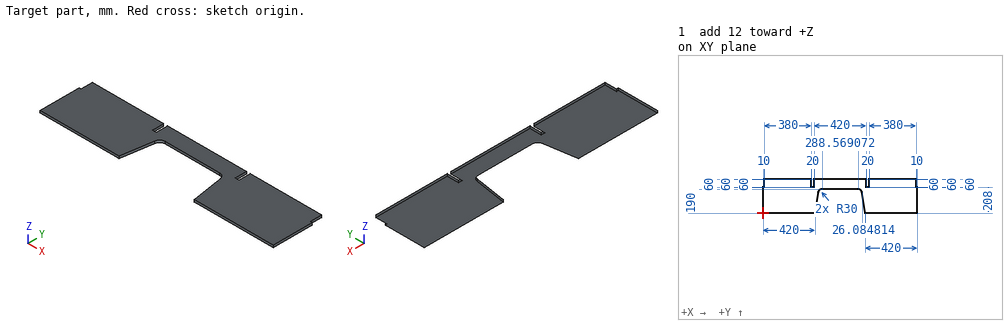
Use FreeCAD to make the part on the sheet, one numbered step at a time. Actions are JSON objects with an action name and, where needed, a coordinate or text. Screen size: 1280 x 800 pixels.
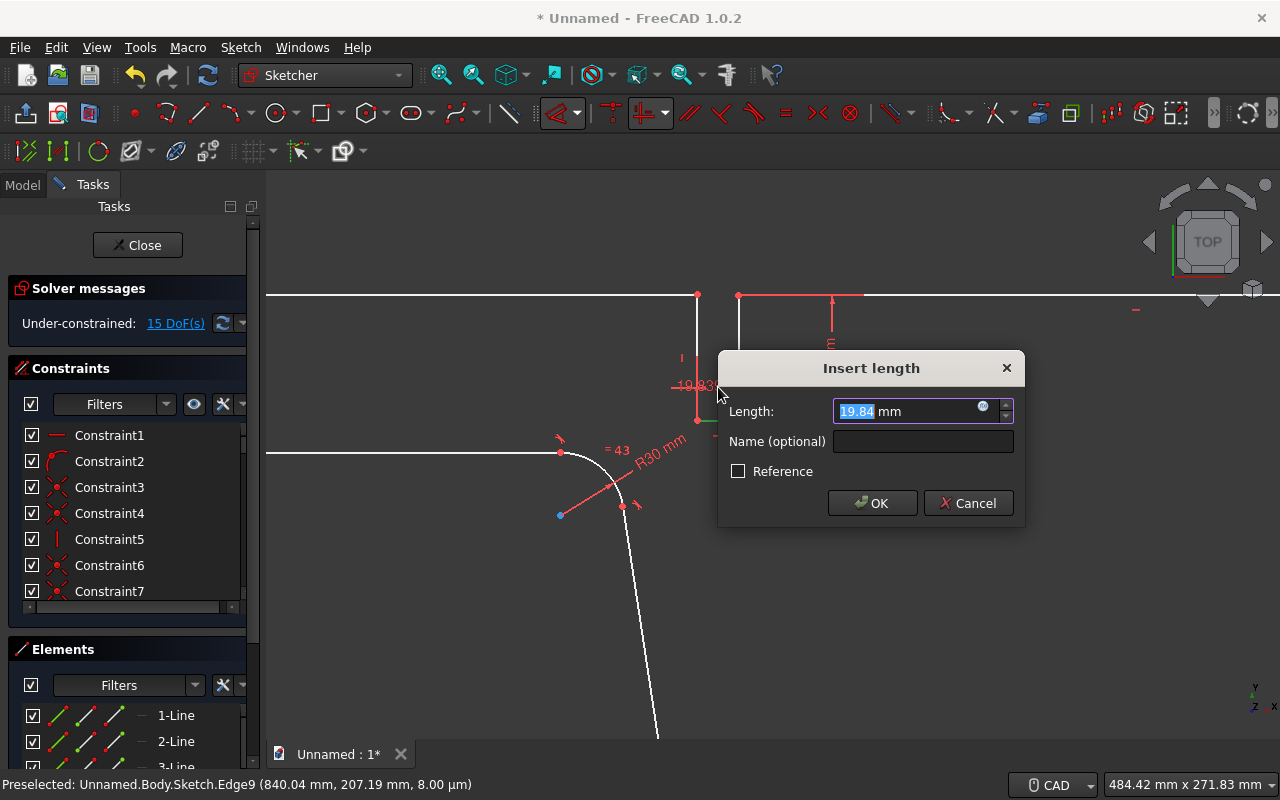
{"action": "type", "text": "20"}
{"action": "key", "text": "Return"}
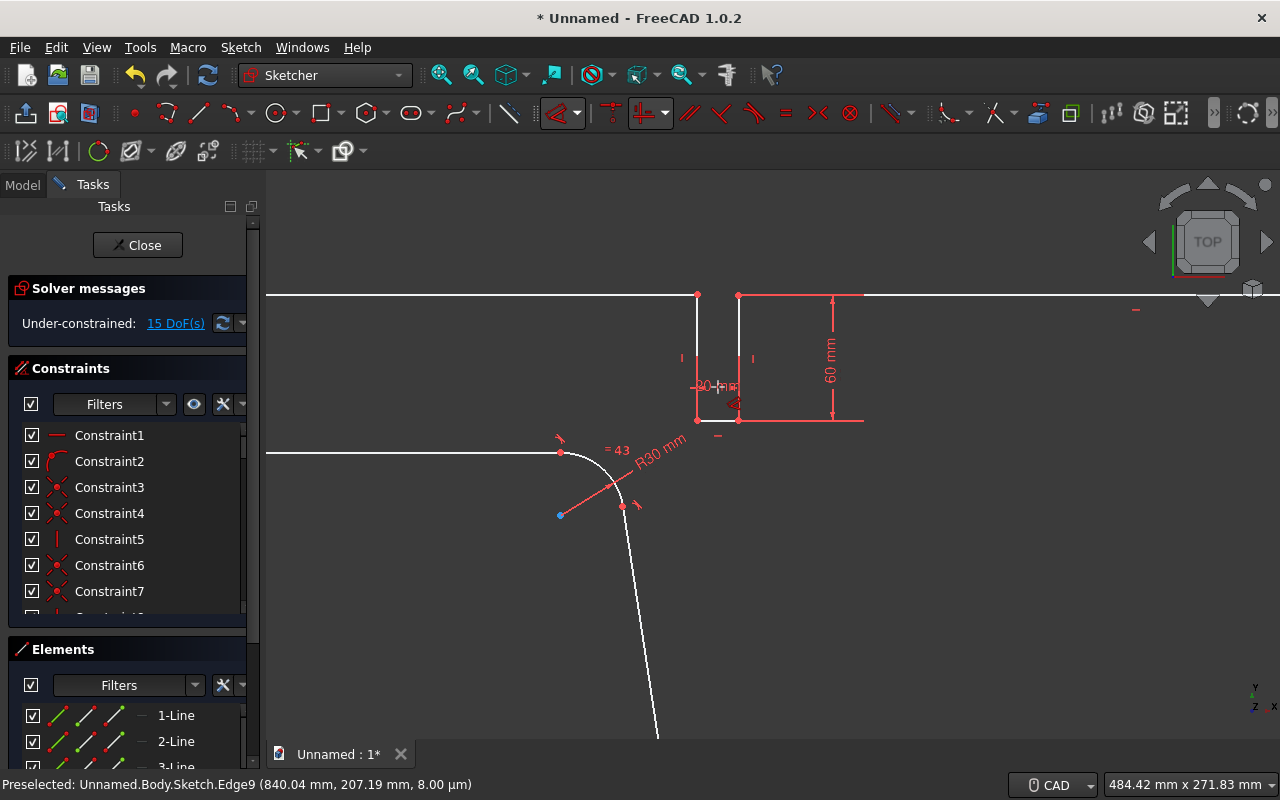
{"action": "left_click", "coordinate": [697, 383]}
{"action": "left_click", "coordinate": [663, 358]}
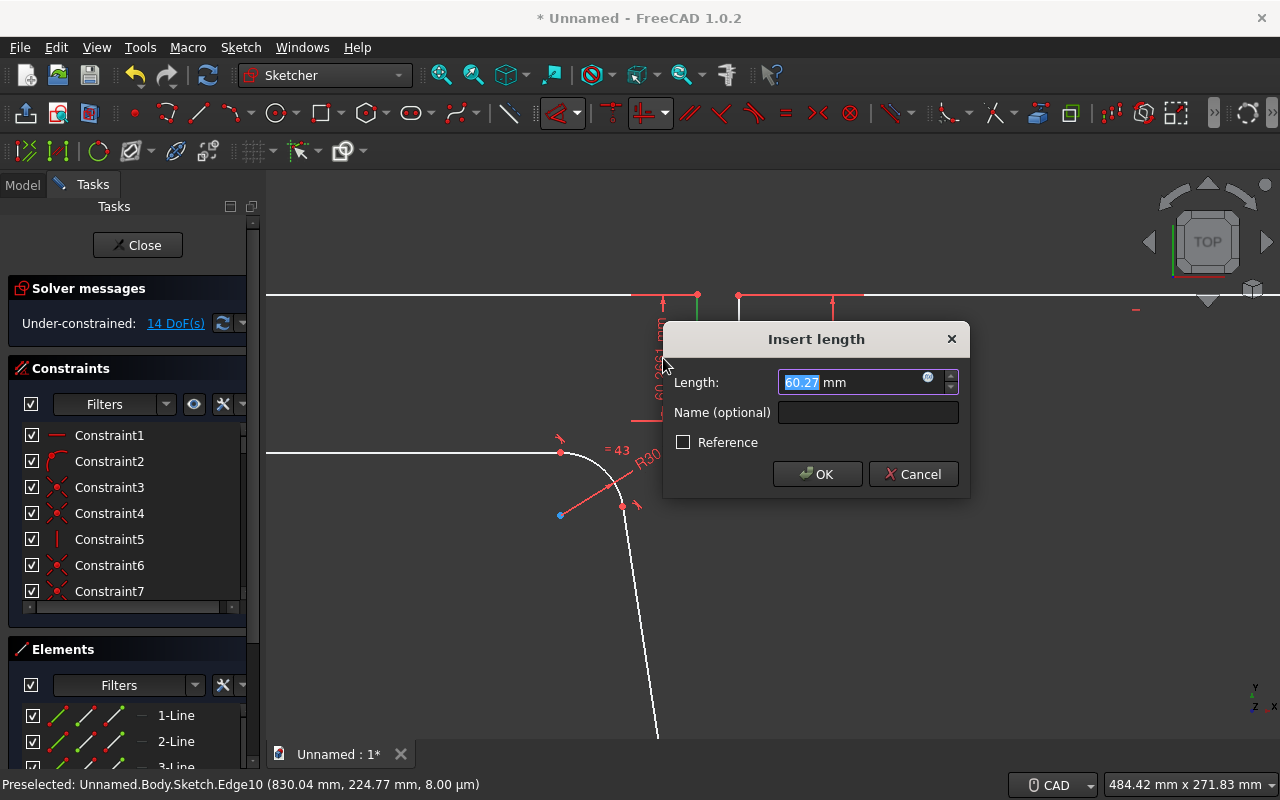
{"action": "type", "text": "60"}
{"action": "key", "text": "Return"}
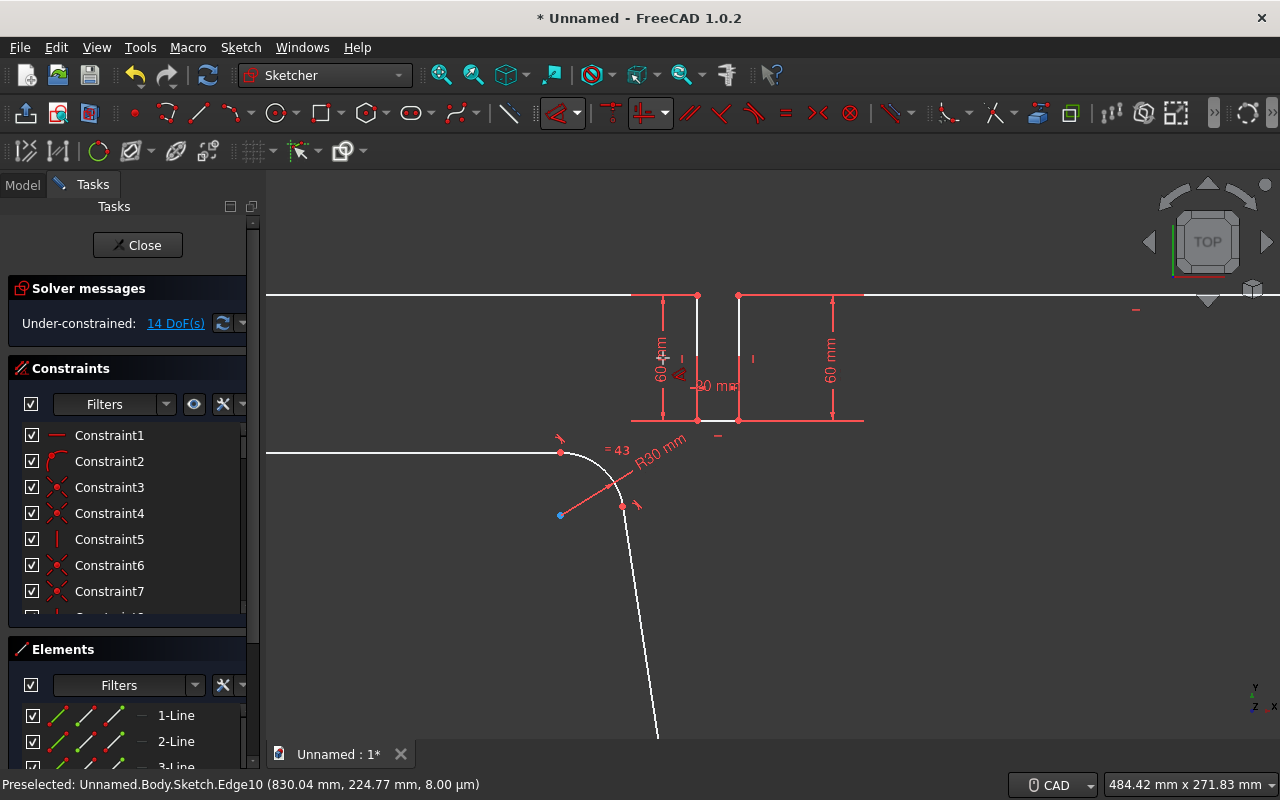
{"action": "scroll", "coordinate": [851, 415], "scroll_direction": "down", "scroll_amount": 7}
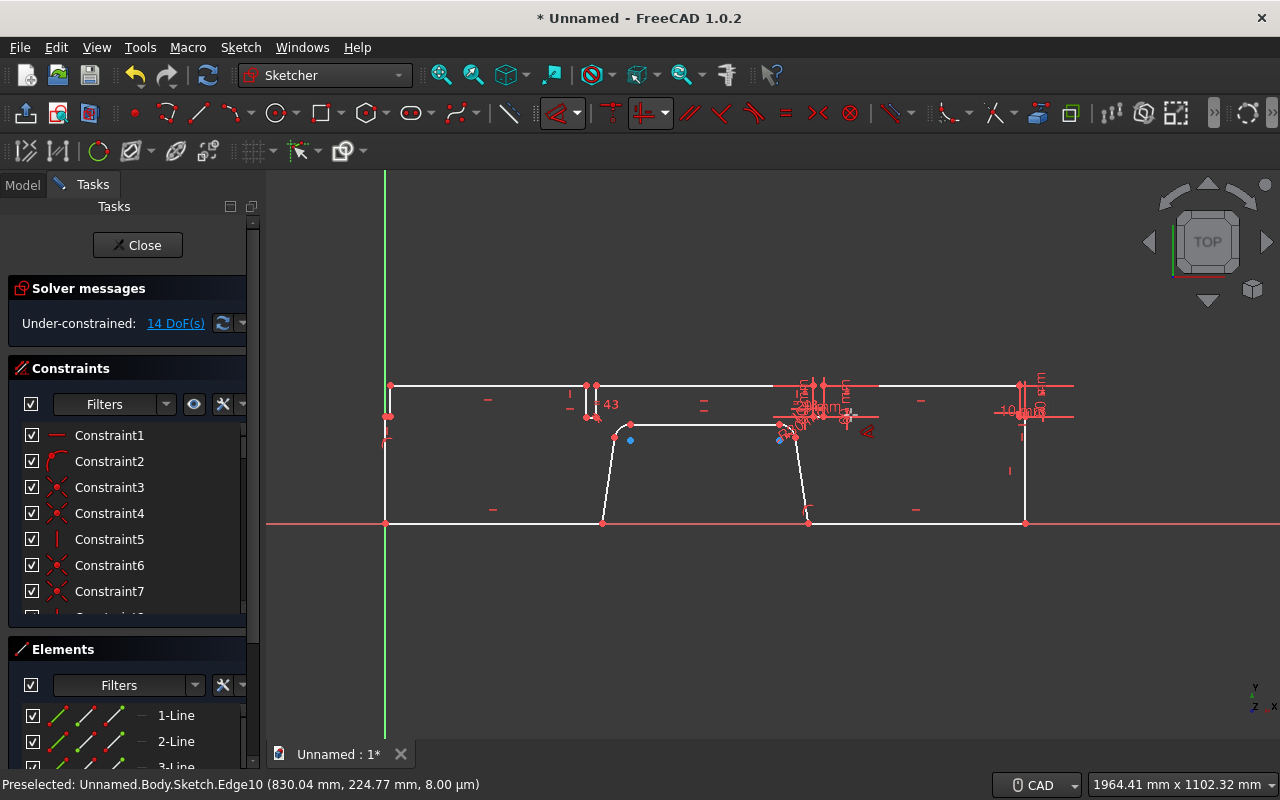
{"action": "scroll", "coordinate": [596, 395], "scroll_direction": "up", "scroll_amount": 2}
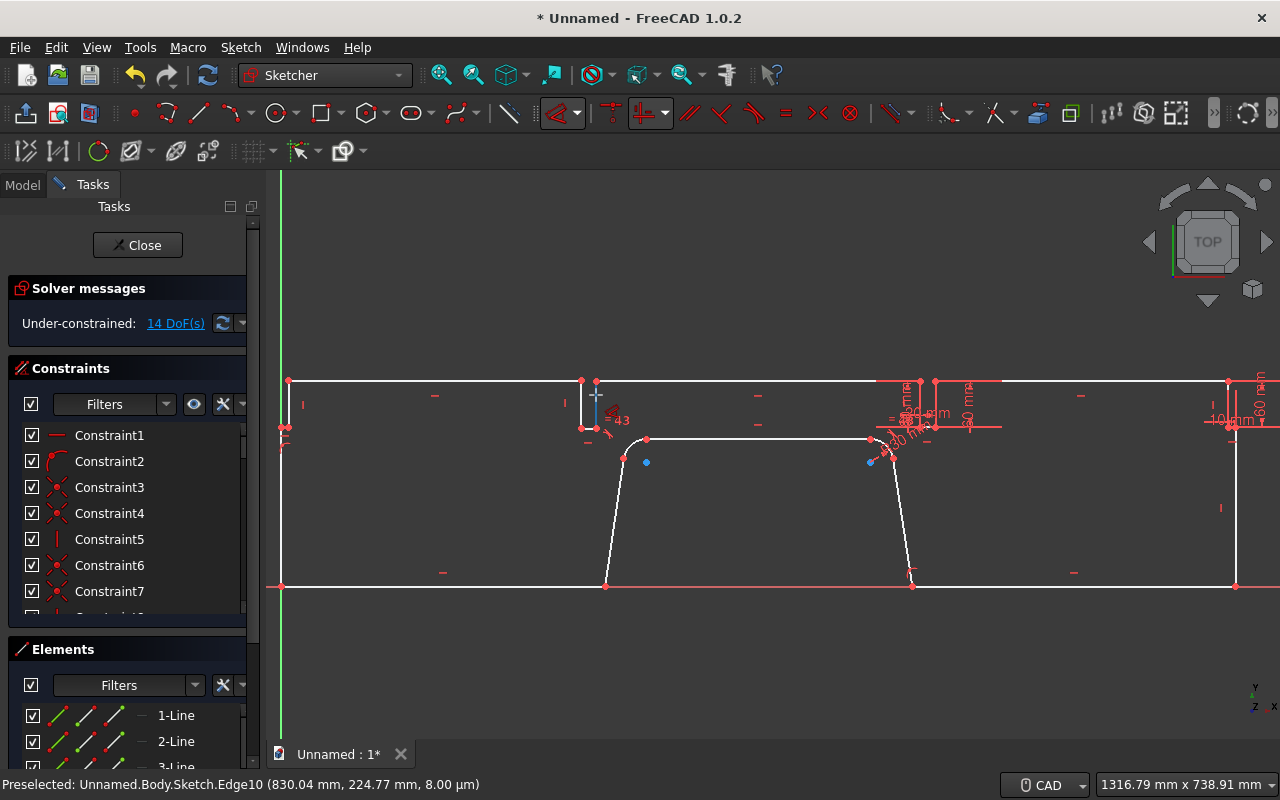
{"action": "left_click", "coordinate": [596, 395]}
{"action": "left_click", "coordinate": [562, 405]}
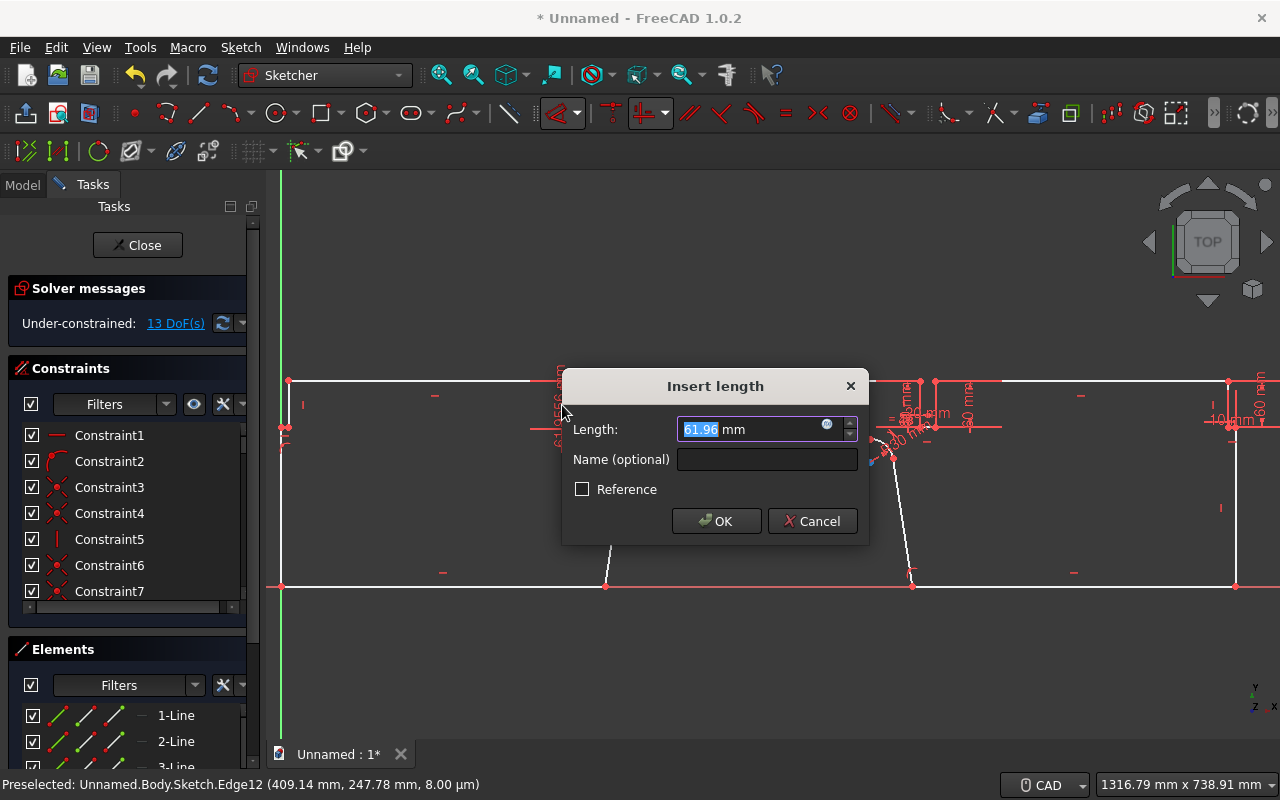
{"action": "type", "text": "60"}
{"action": "key", "text": "Return"}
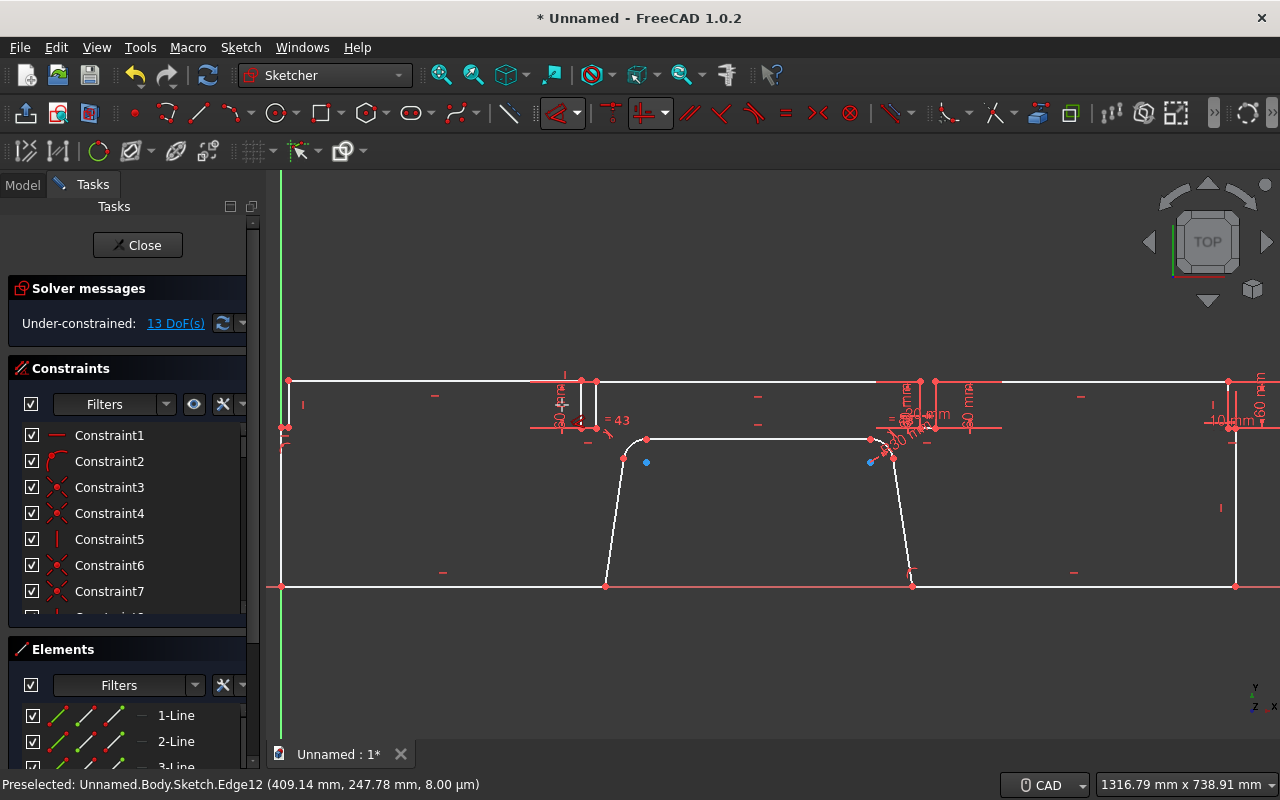
{"action": "scroll", "coordinate": [589, 428], "scroll_direction": "up", "scroll_amount": 5}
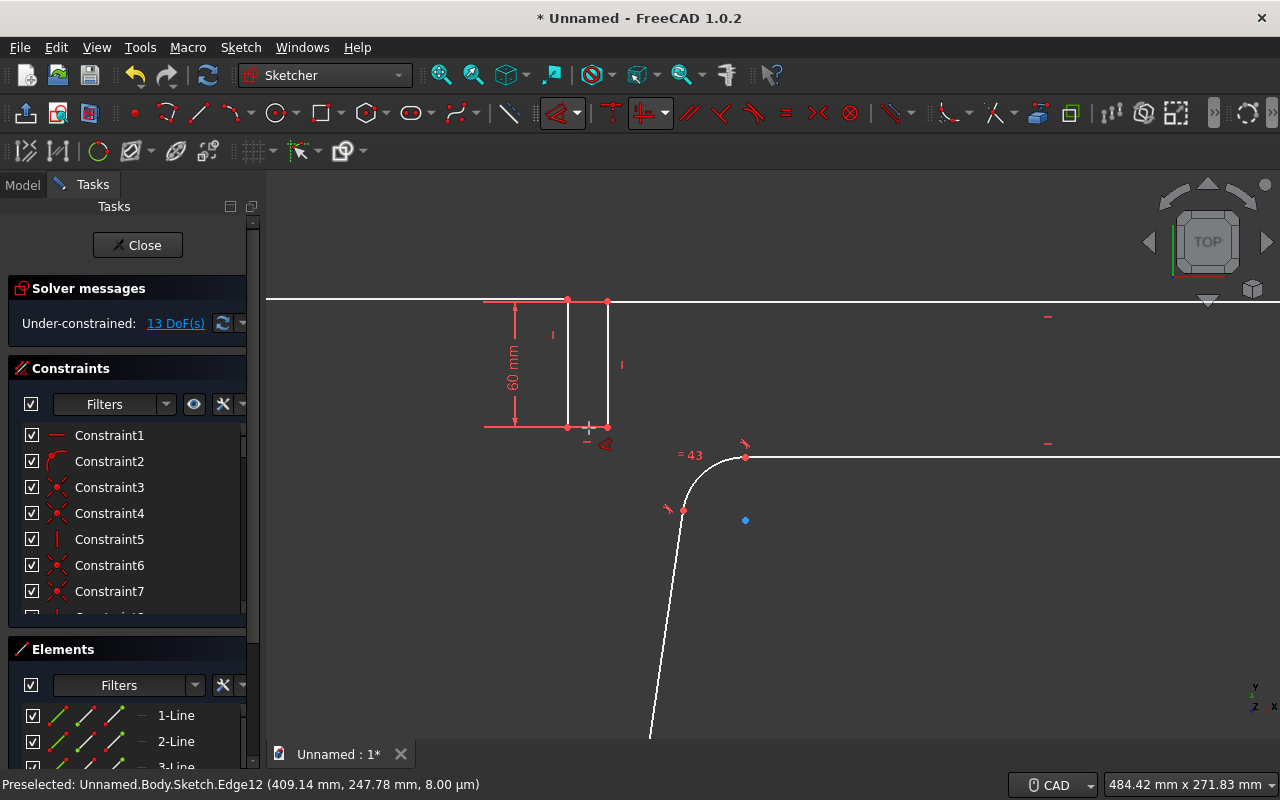
{"action": "left_click", "coordinate": [588, 427]}
{"action": "left_click", "coordinate": [588, 393]}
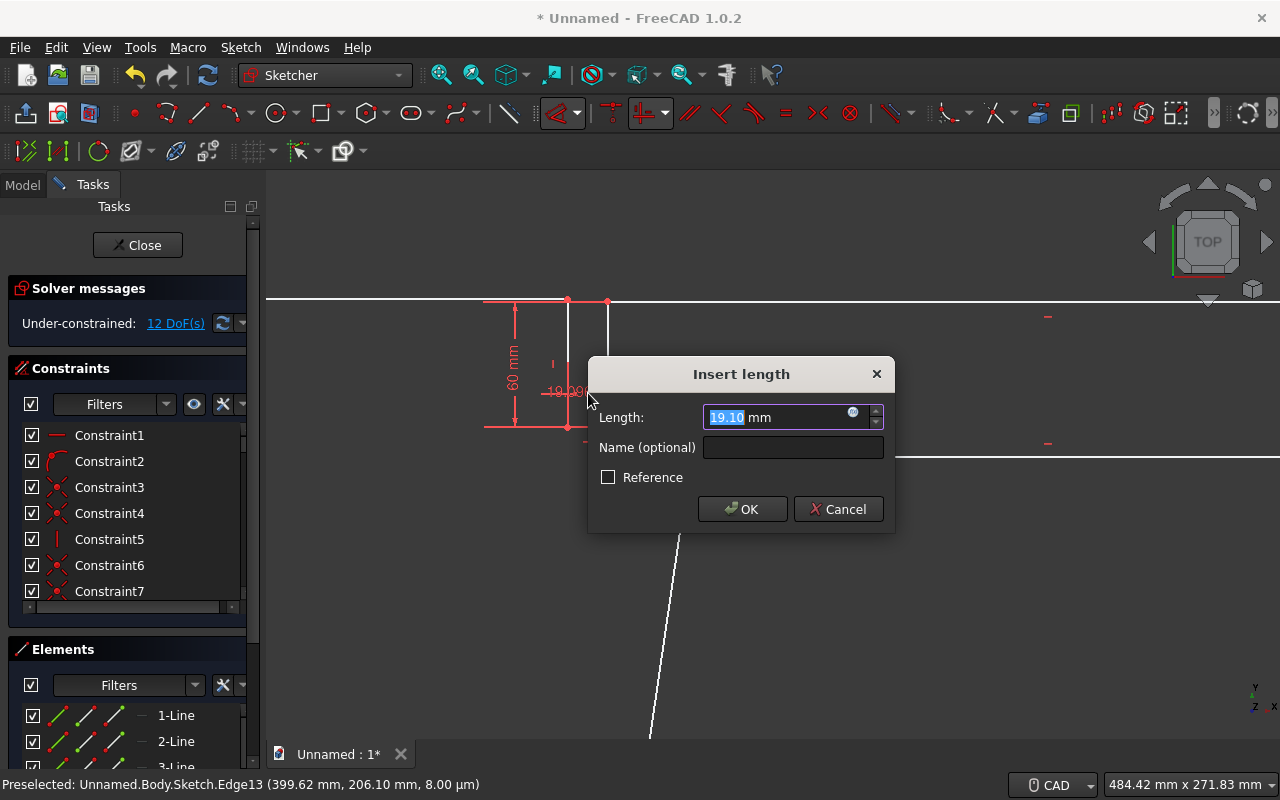
{"action": "type", "text": "20"}
{"action": "key", "text": "Return"}